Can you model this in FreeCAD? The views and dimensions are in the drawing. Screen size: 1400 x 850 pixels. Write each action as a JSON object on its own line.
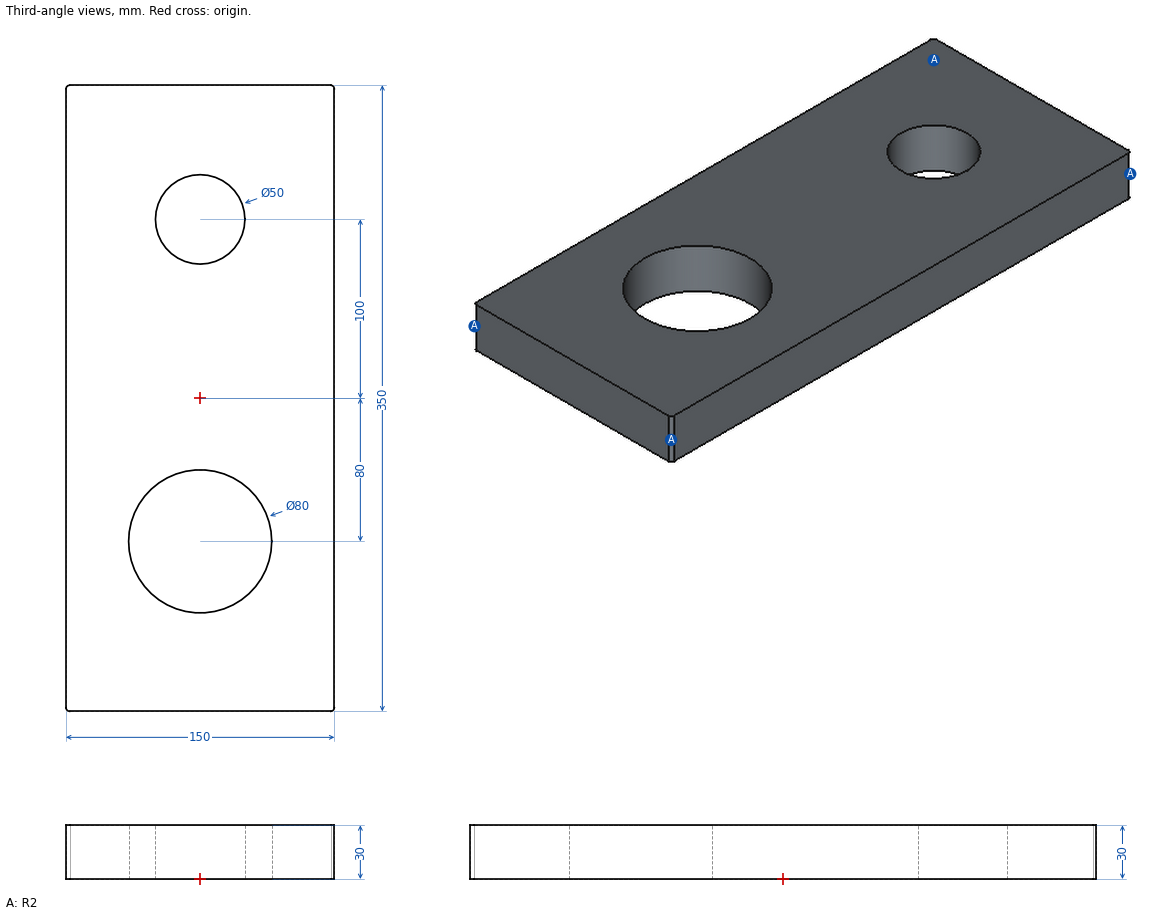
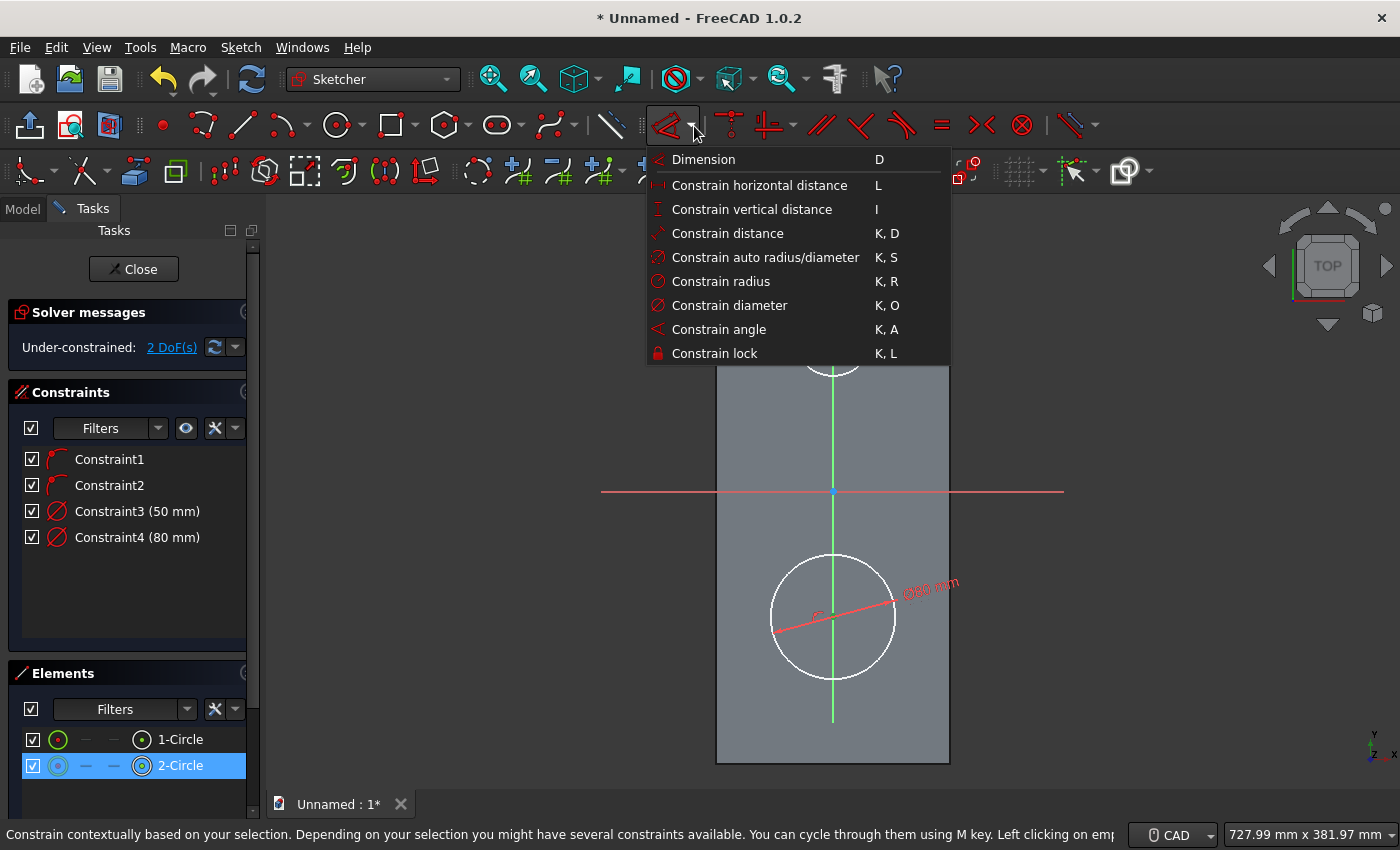
{"action": "left_click", "coordinate": [799, 209]}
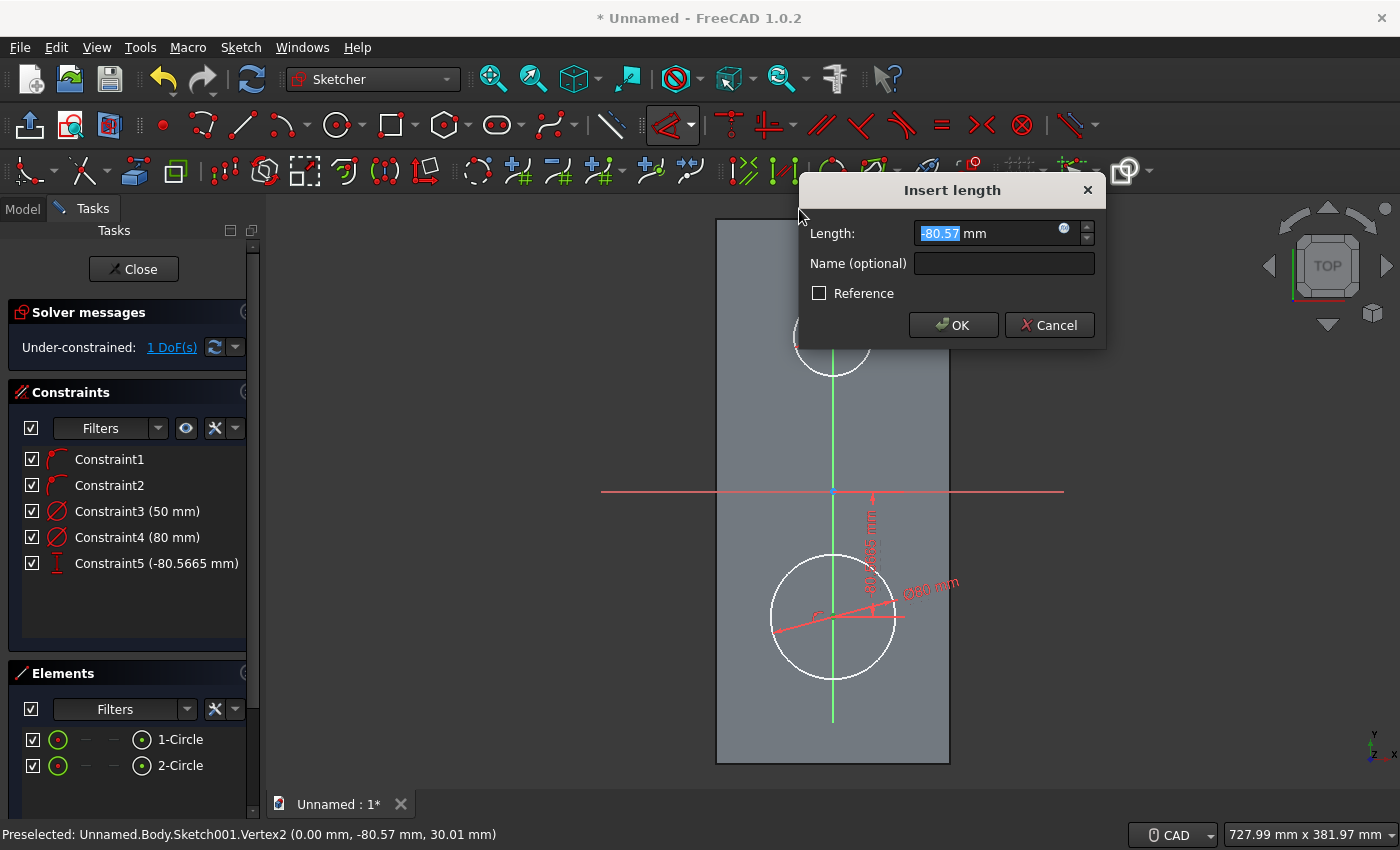
{"action": "type", "text": "-80"}
{"action": "key", "text": "Return"}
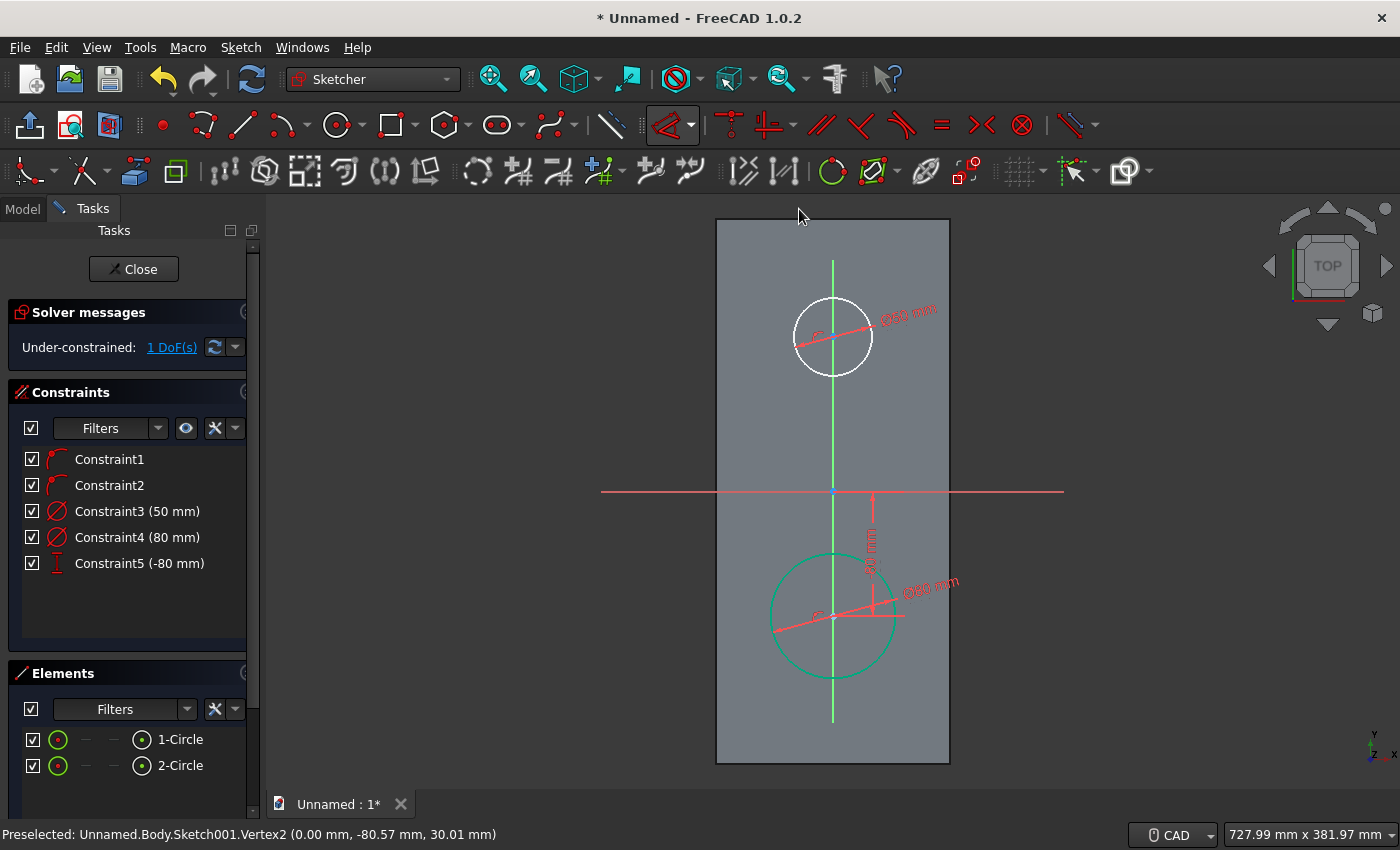
{"action": "left_click", "coordinate": [833, 337]}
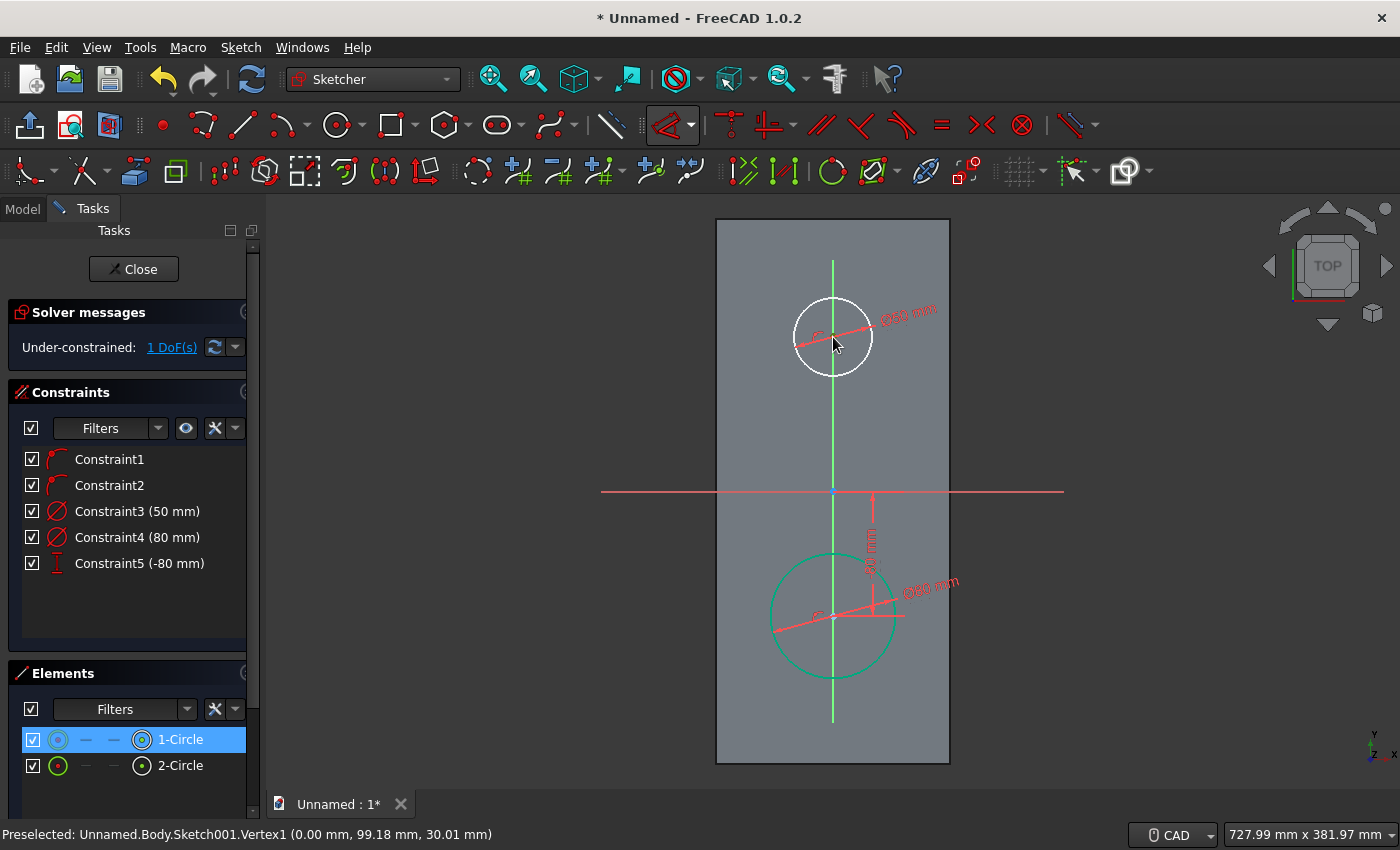
{"action": "key", "text": "i"}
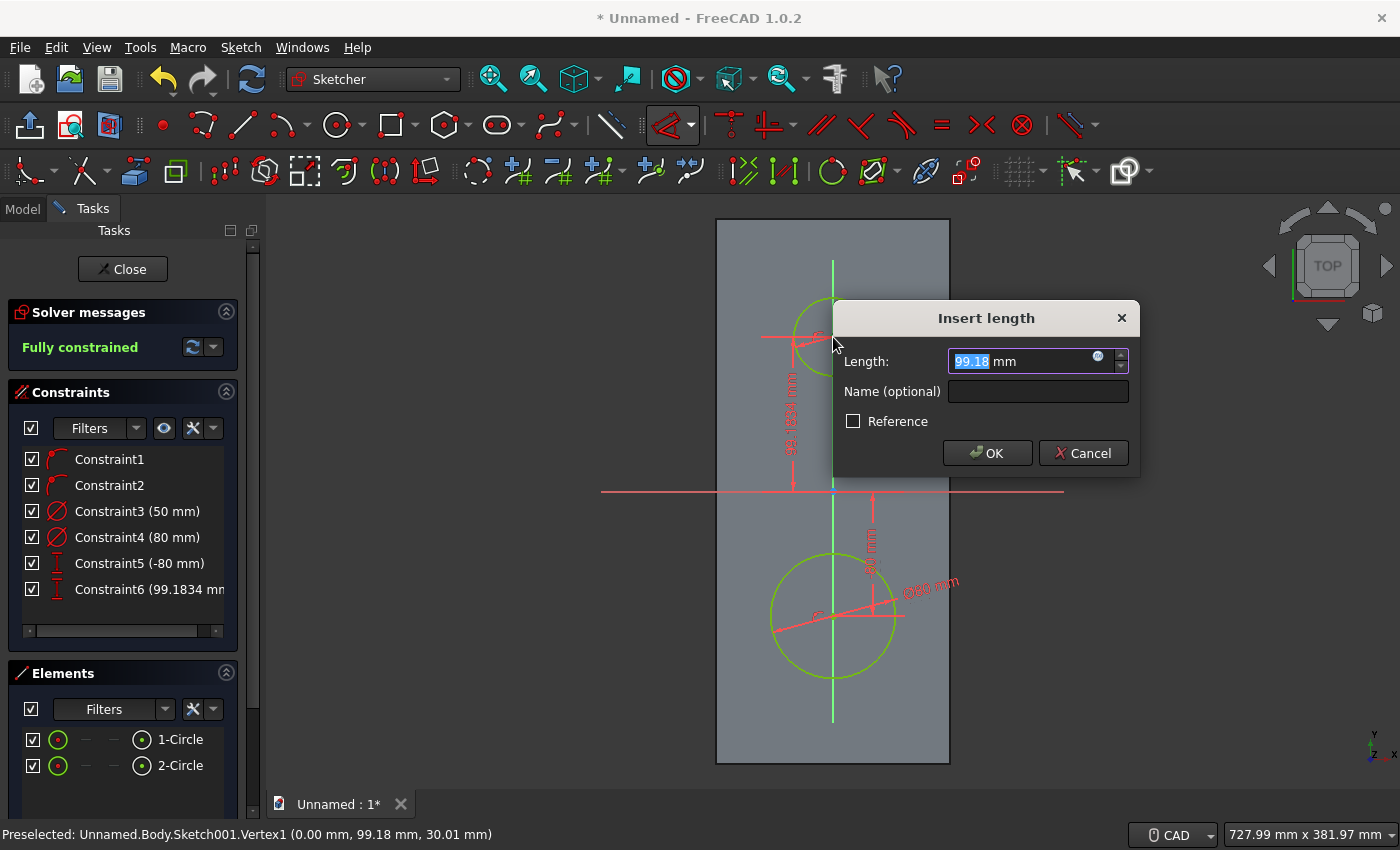
{"action": "type", "text": "100"}
{"action": "key", "text": "Return"}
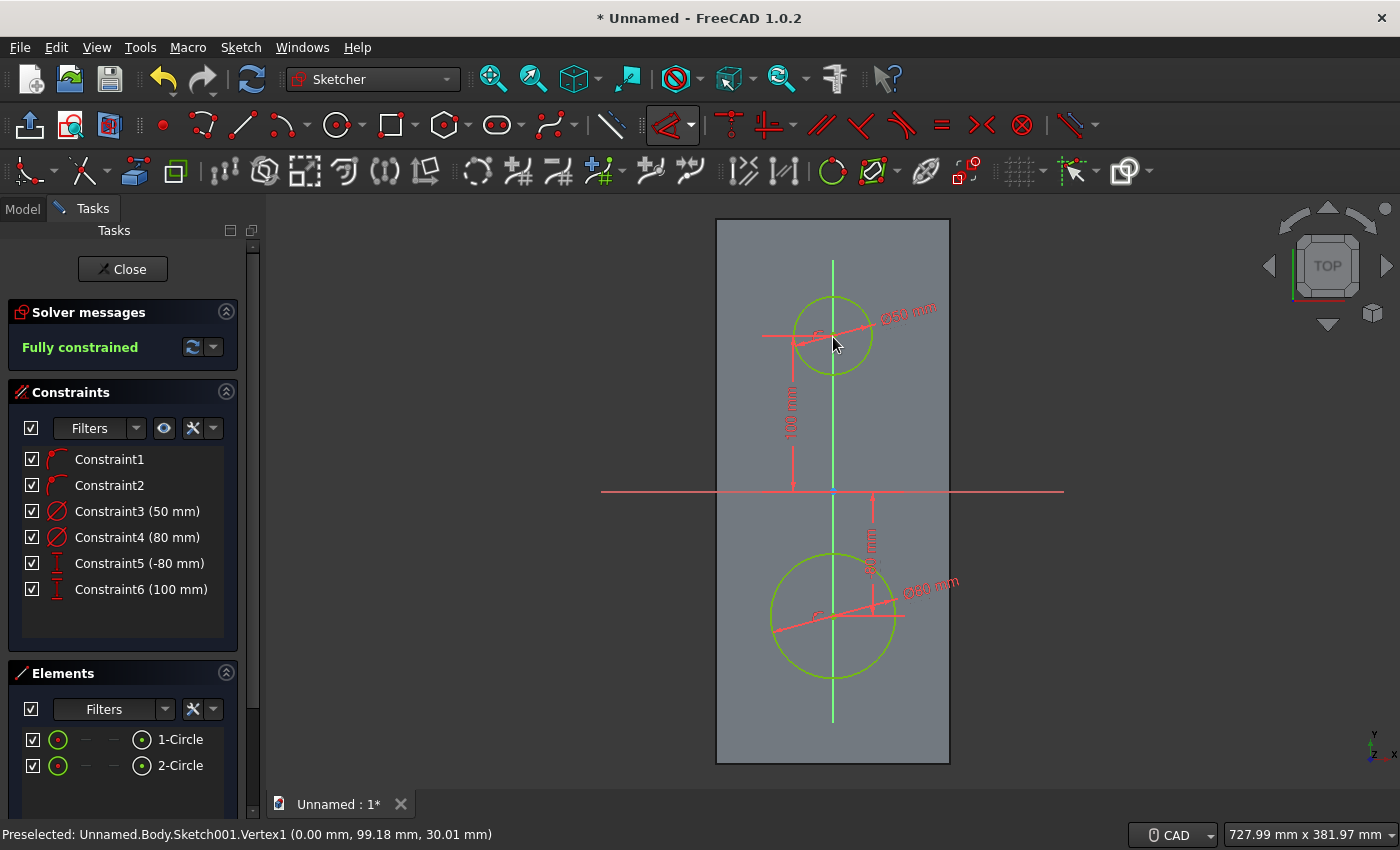
{"action": "left_click", "coordinate": [123, 269]}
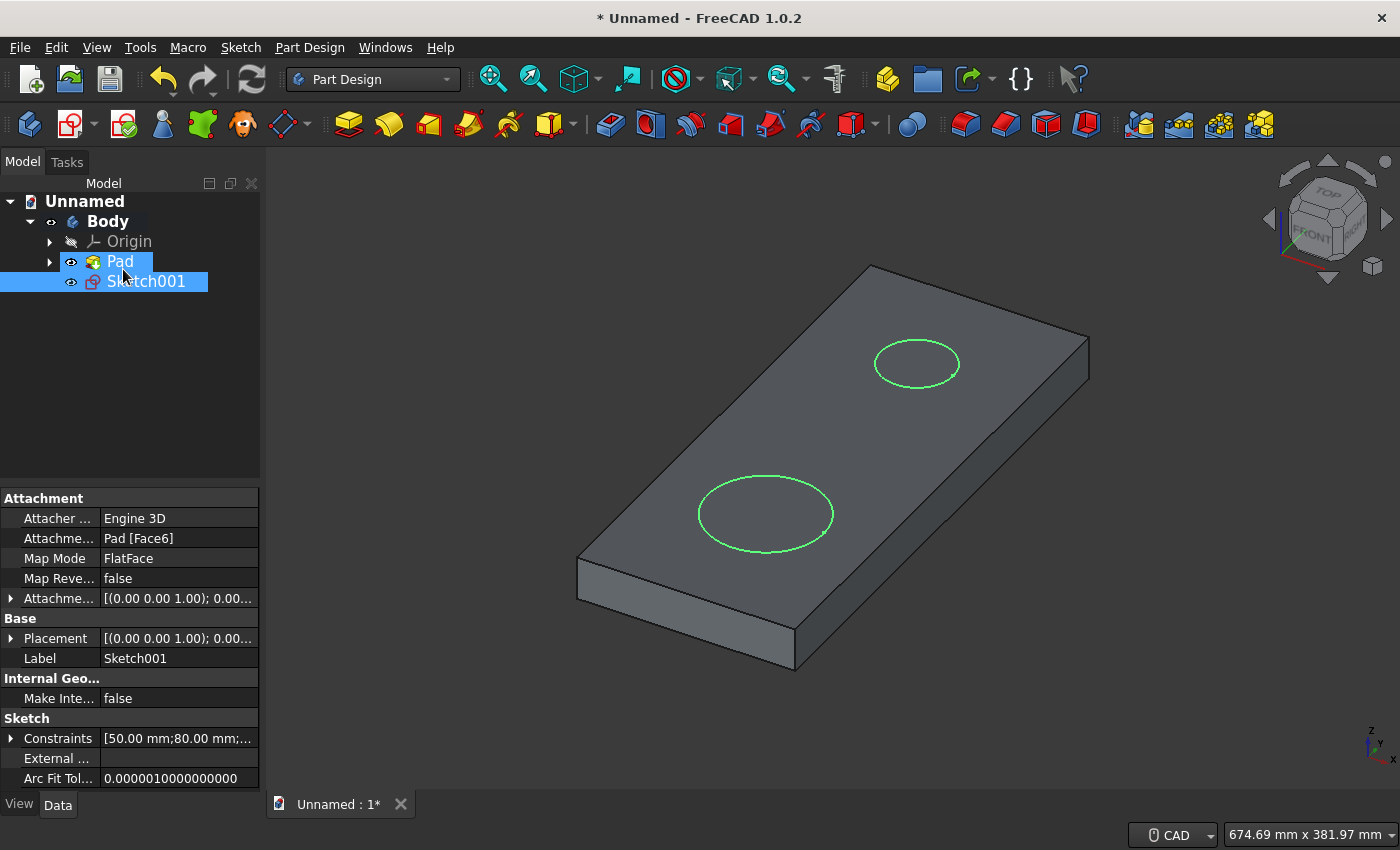
{"action": "left_click", "coordinate": [612, 124]}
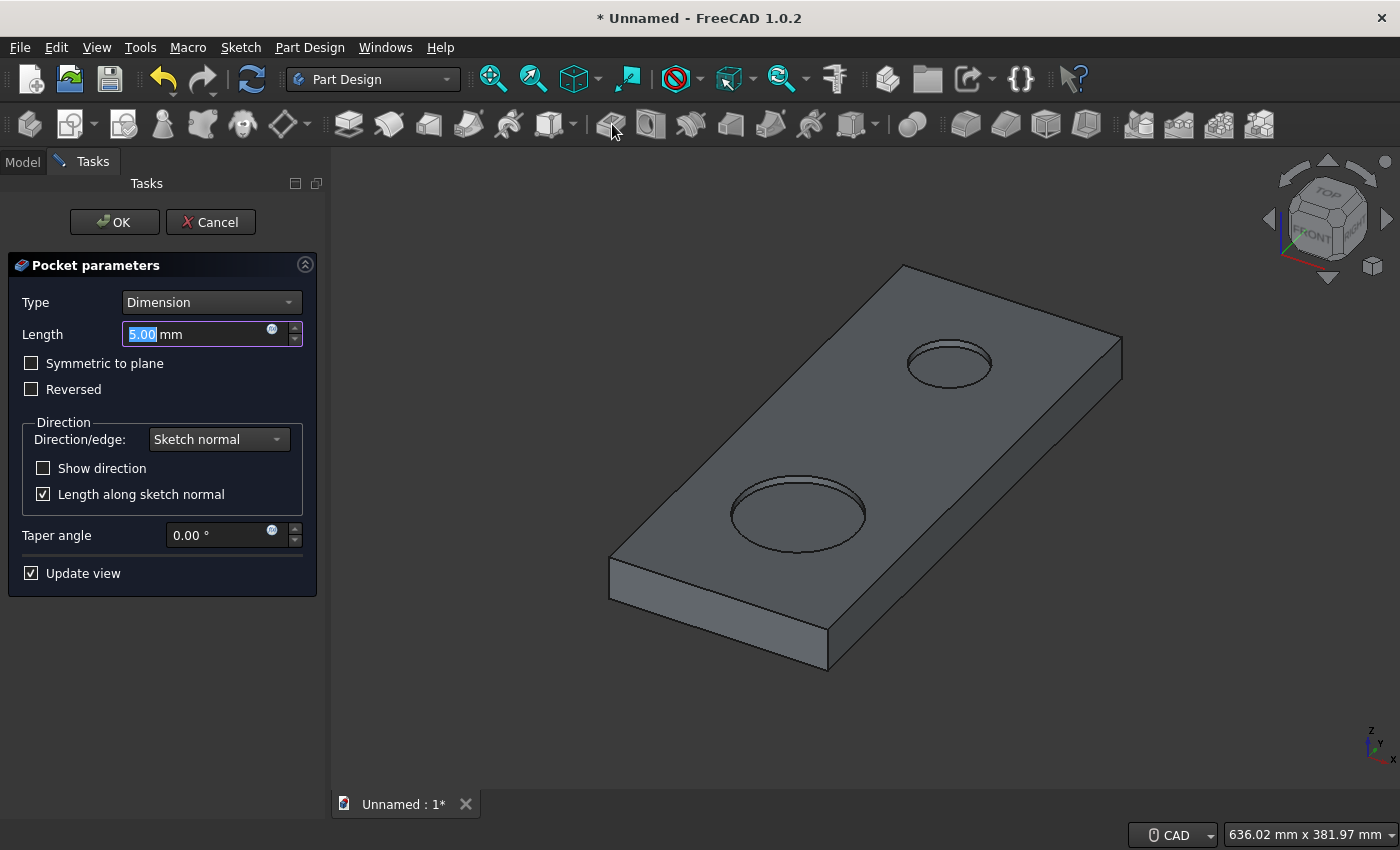
{"action": "type", "text": "30"}
{"action": "key", "text": "Tab"}